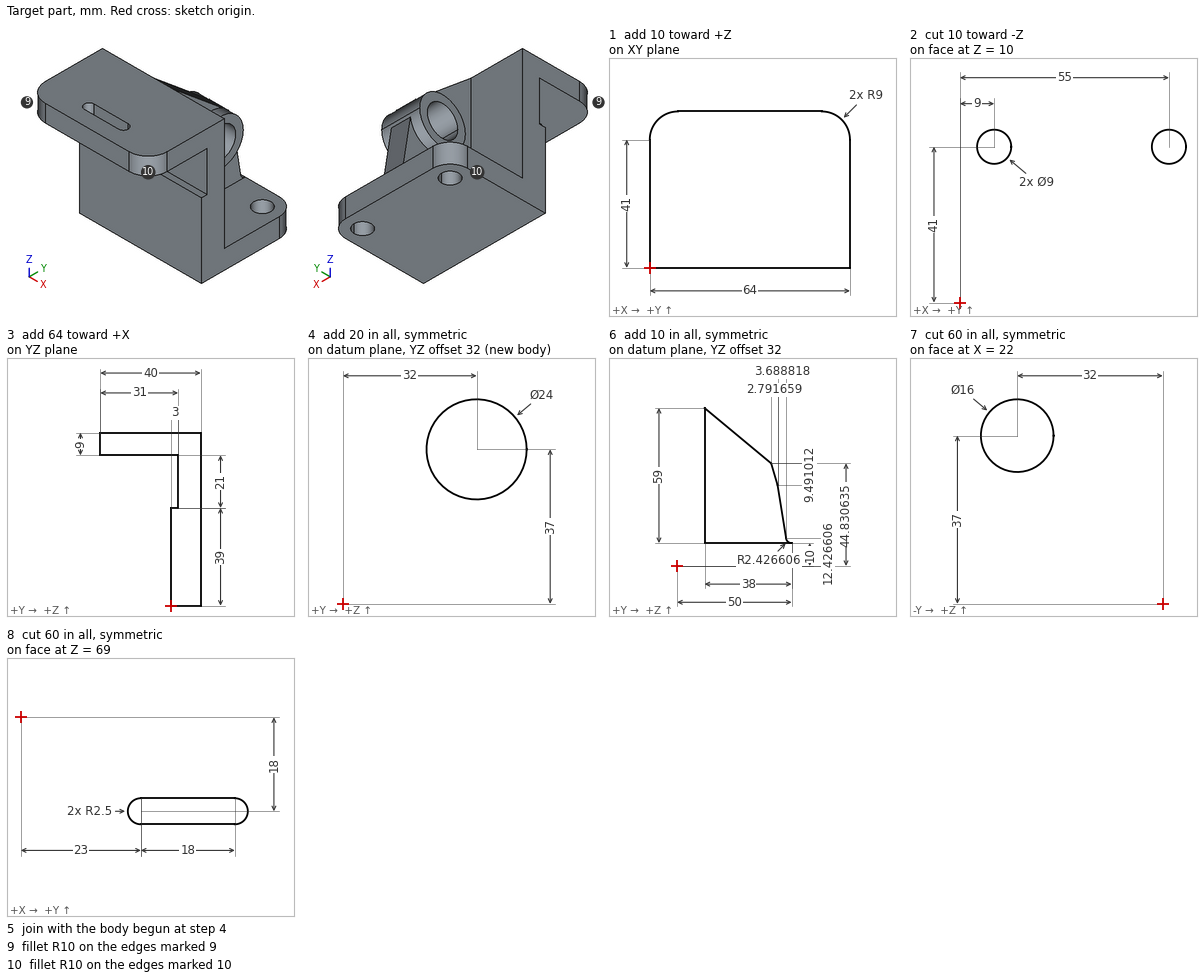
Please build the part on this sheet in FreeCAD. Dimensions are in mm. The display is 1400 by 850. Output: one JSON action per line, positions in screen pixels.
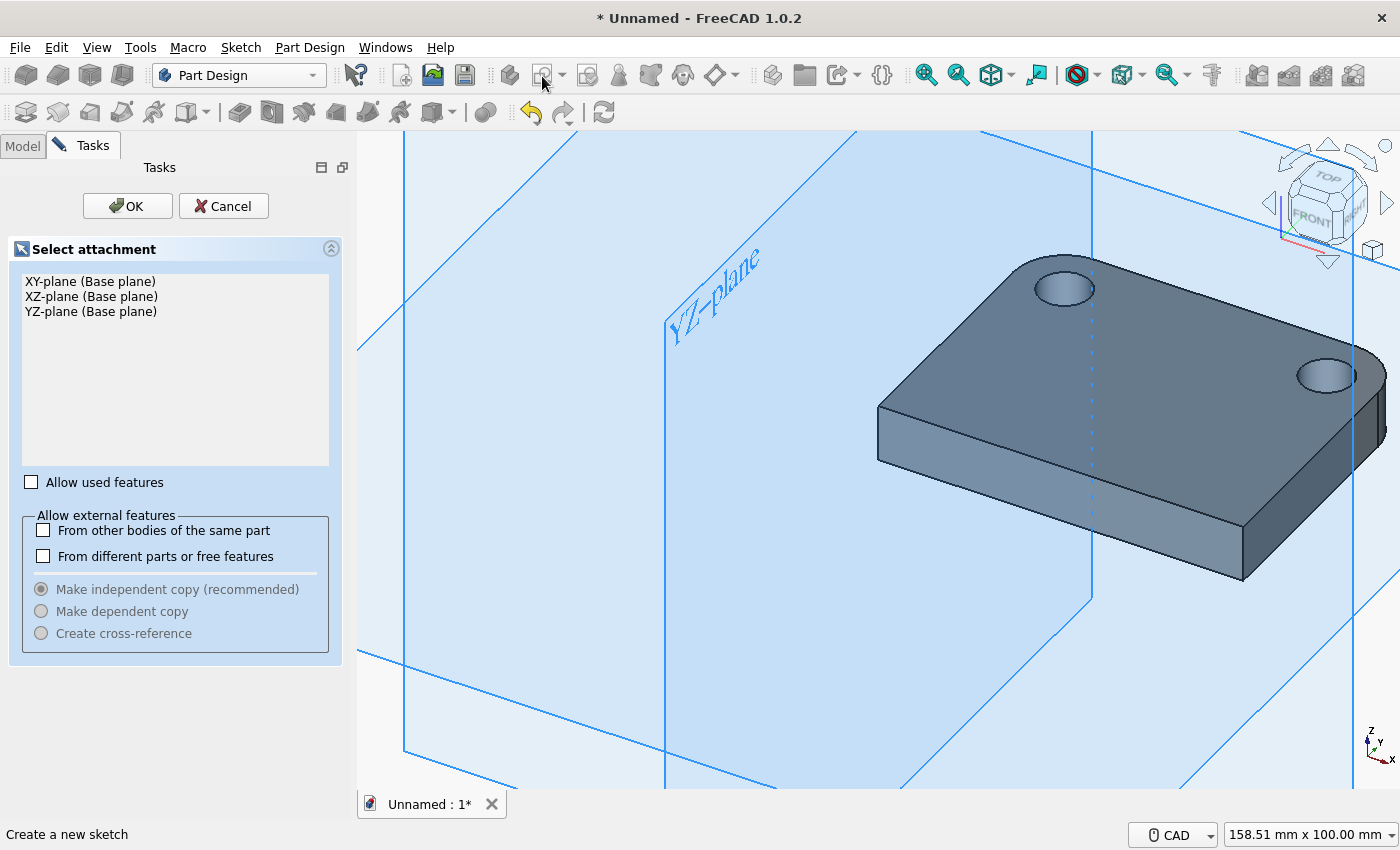
{"action": "left_click", "coordinate": [82, 312]}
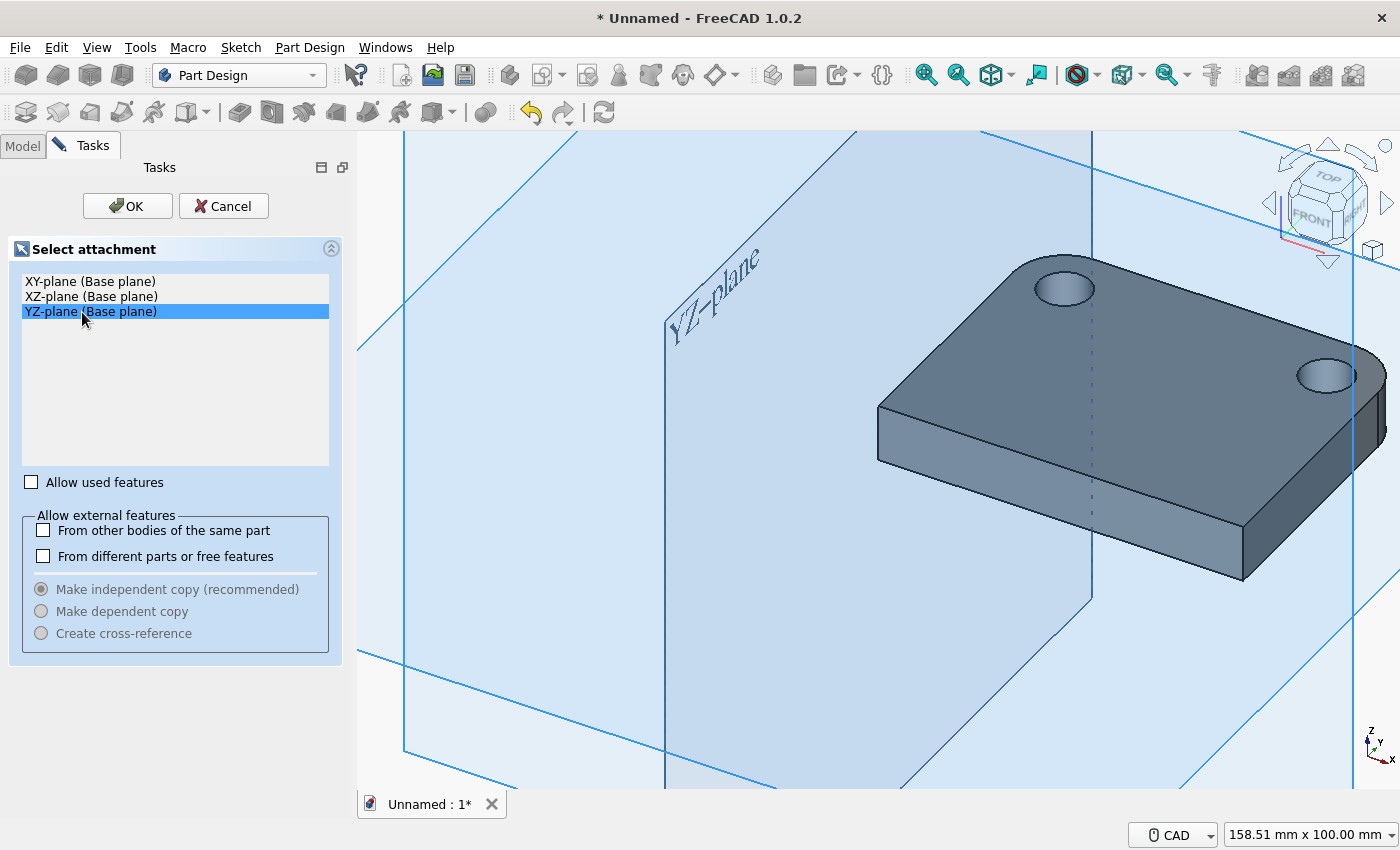
{"action": "left_click", "coordinate": [128, 206]}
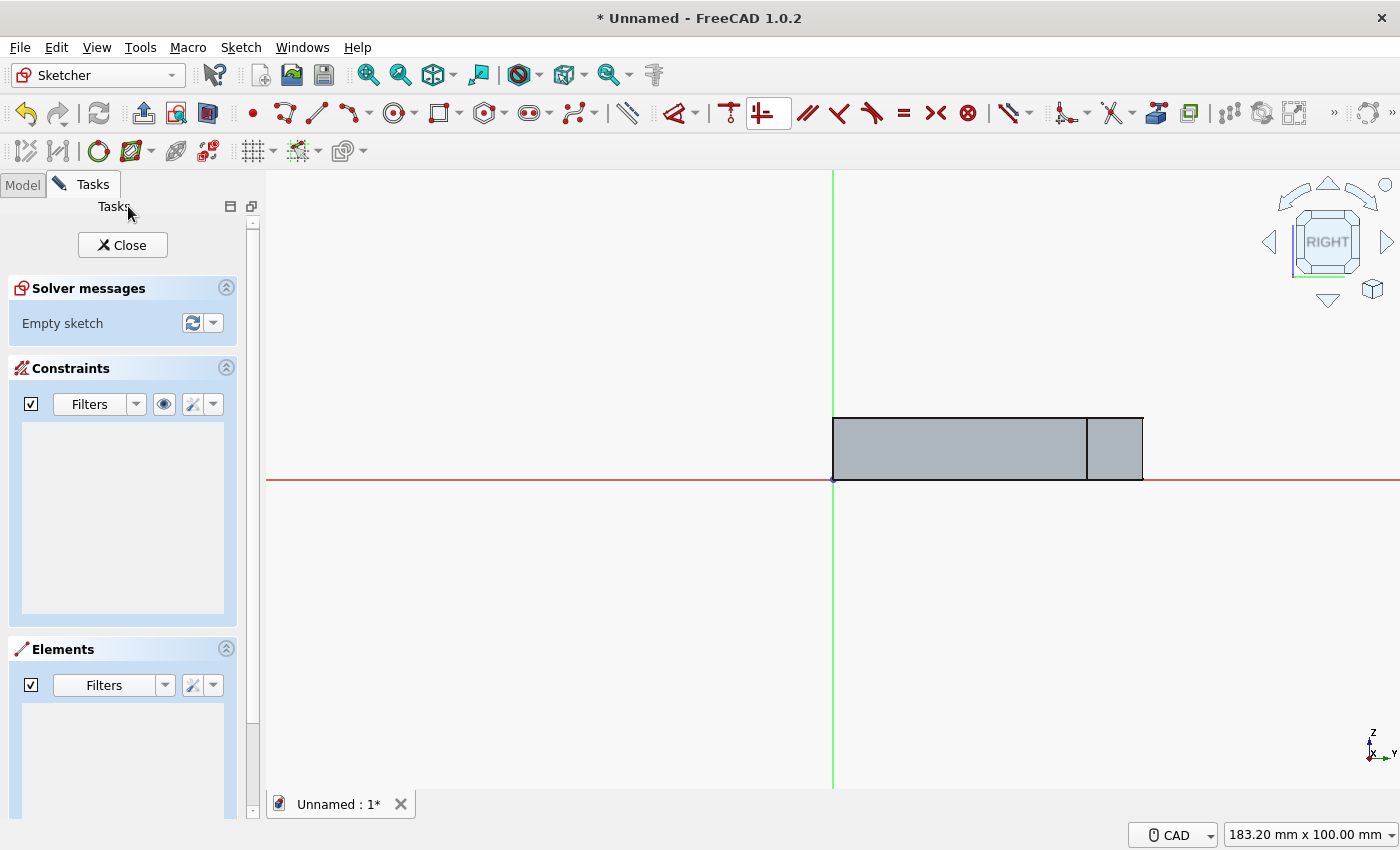
{"action": "left_click", "coordinate": [208, 114]}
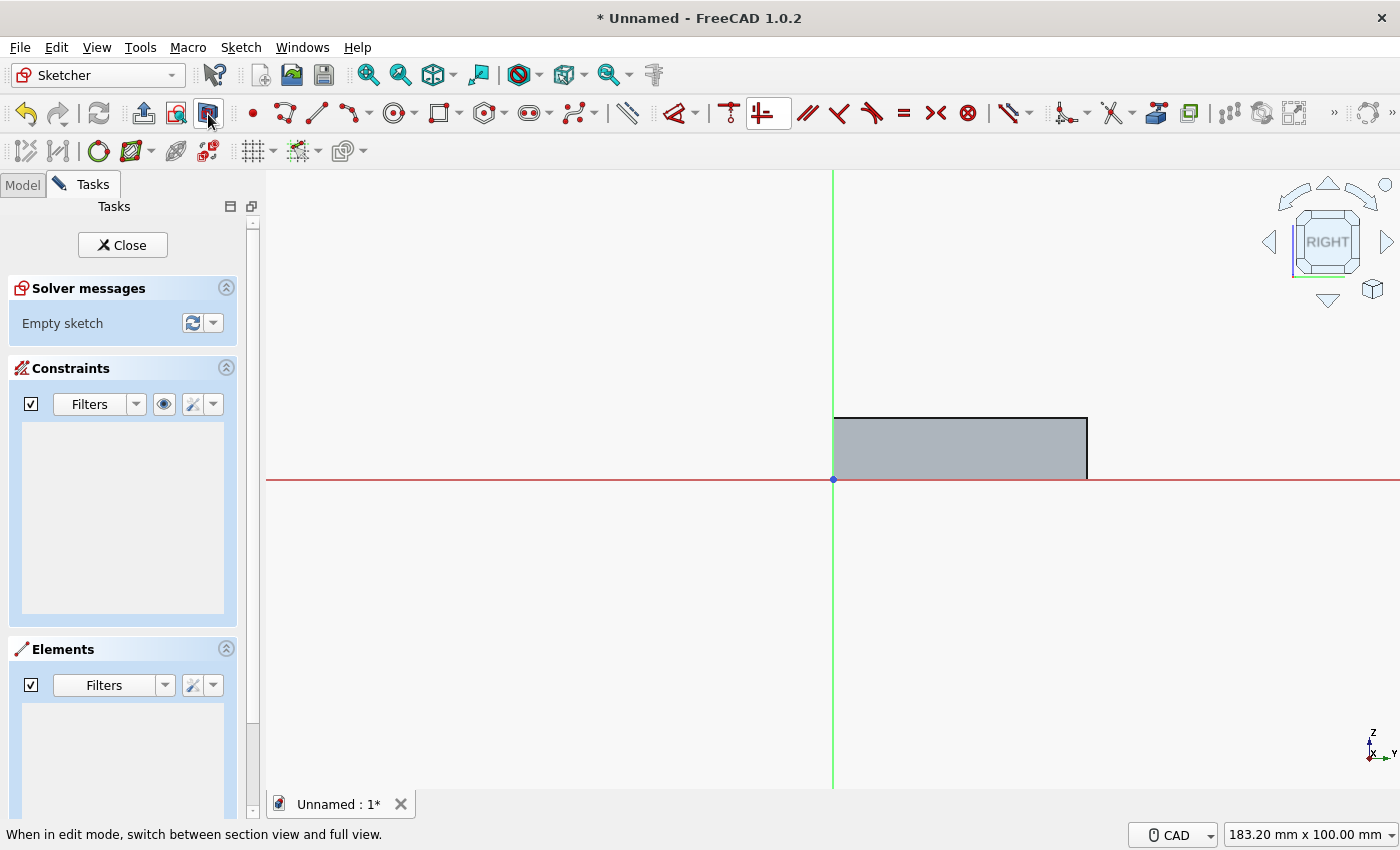
{"action": "scroll", "coordinate": [726, 761], "scroll_direction": "down", "scroll_amount": 2}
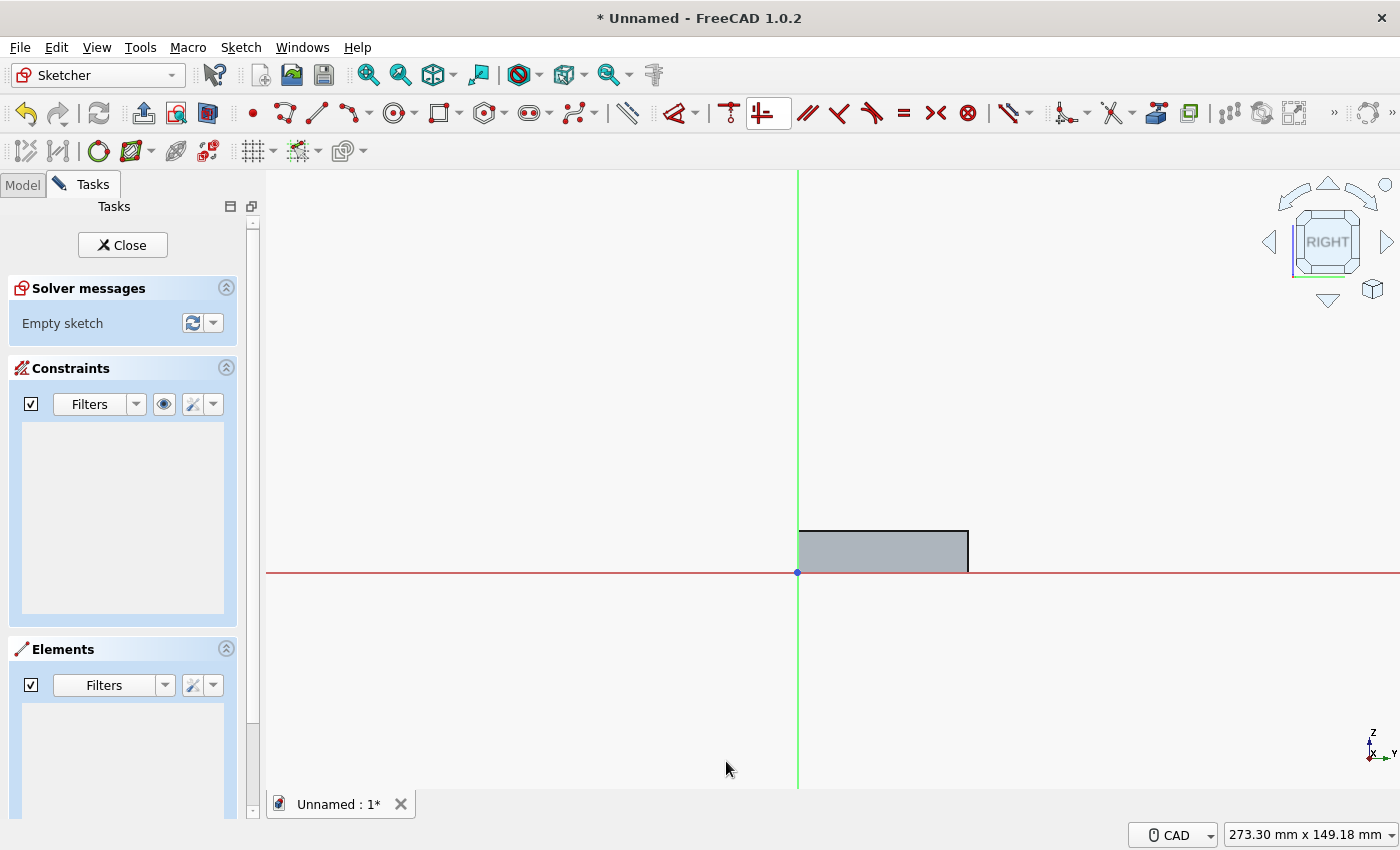
{"action": "scroll", "coordinate": [765, 328], "scroll_direction": "up", "scroll_amount": 2}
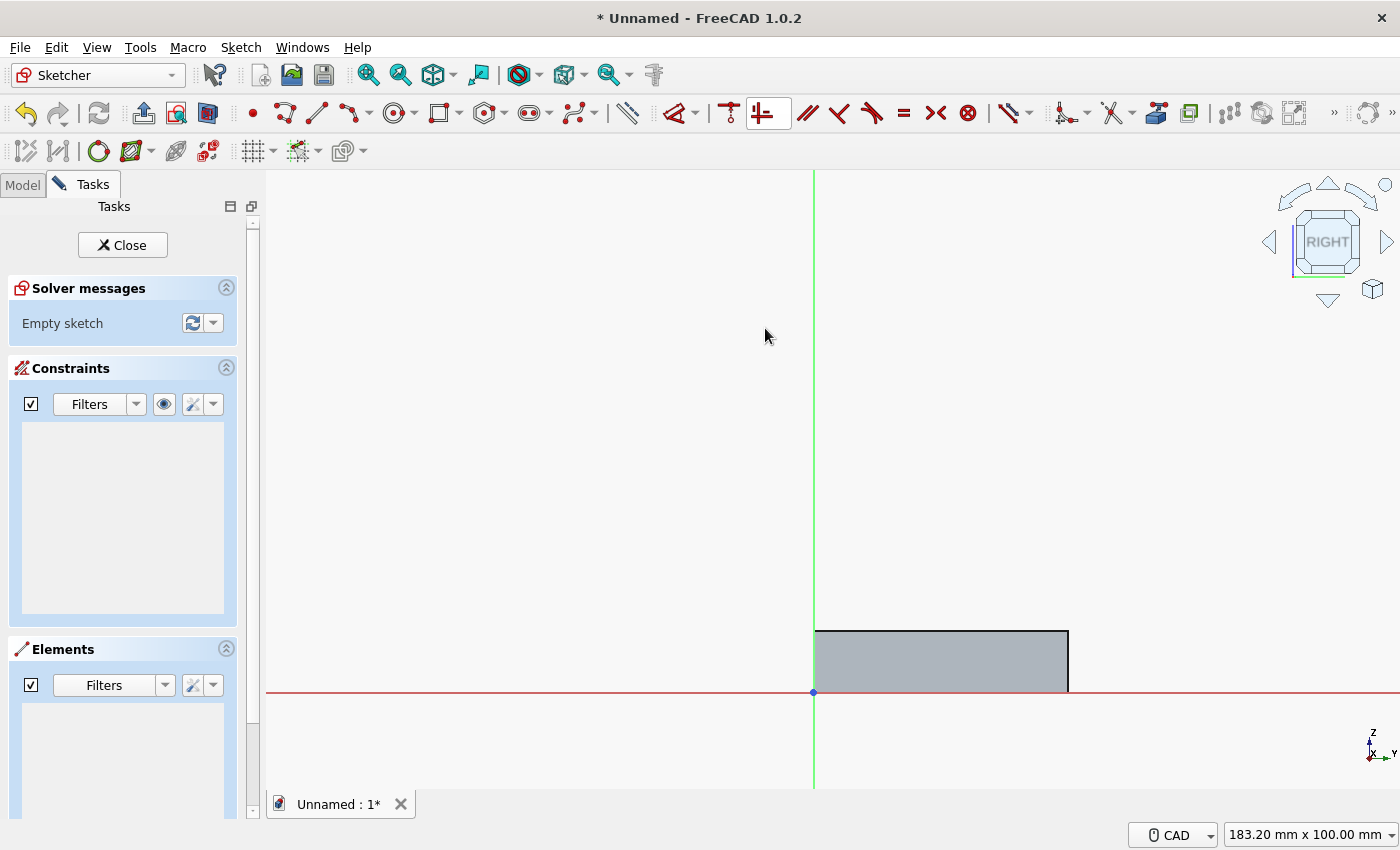
{"action": "left_click", "coordinate": [286, 114]}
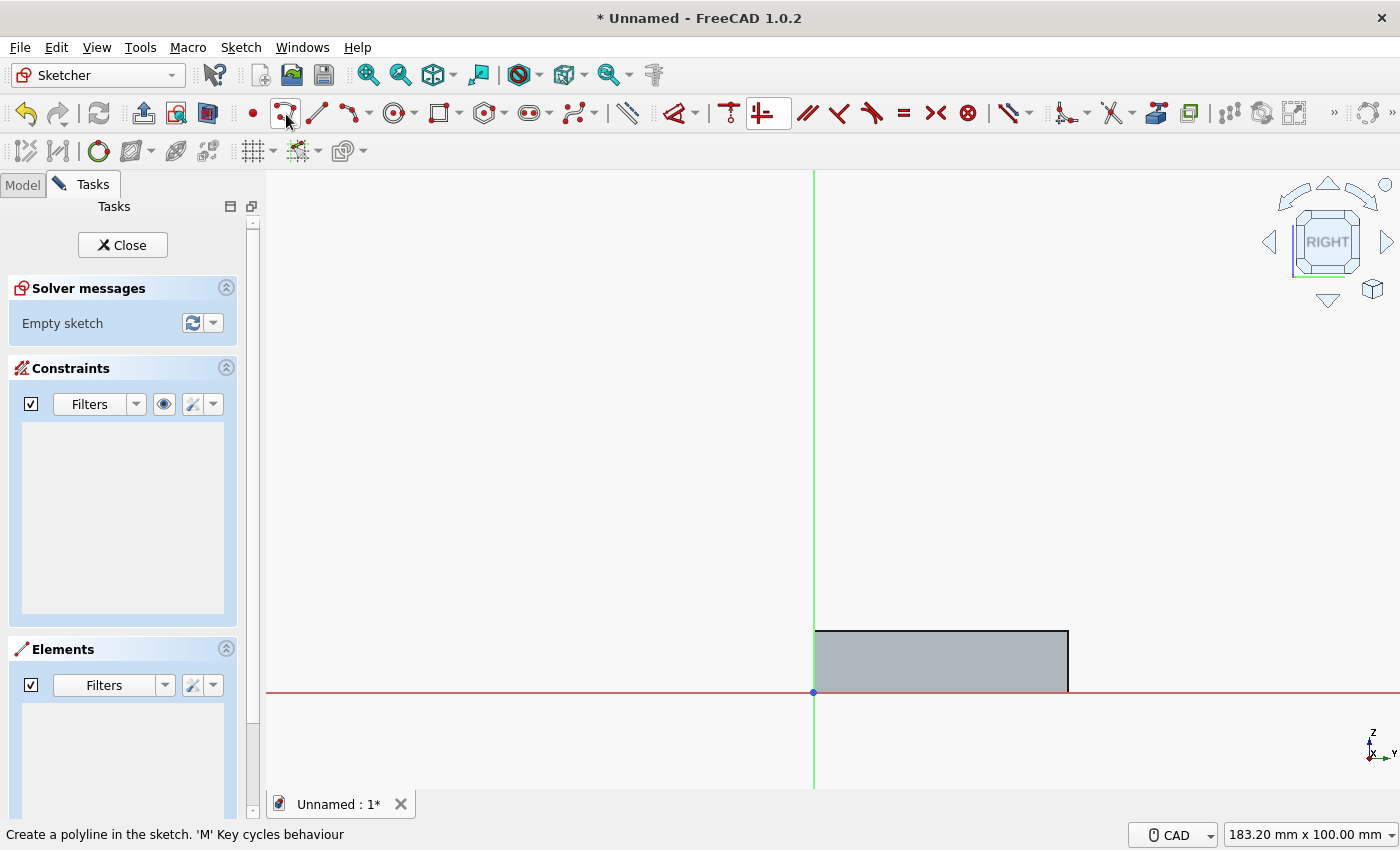
{"action": "left_click", "coordinate": [814, 693]}
{"action": "left_click", "coordinate": [805, 451]}
{"action": "left_click", "coordinate": [832, 451]}
{"action": "left_click", "coordinate": [832, 321]}
{"action": "left_click", "coordinate": [640, 321]}
{"action": "left_click", "coordinate": [640, 266]}
{"action": "left_click", "coordinate": [888, 266]}
{"action": "left_click", "coordinate": [888, 684]}
{"action": "left_click", "coordinate": [814, 693]}
{"action": "key", "text": "Escape"}
{"action": "key", "text": "Escape"}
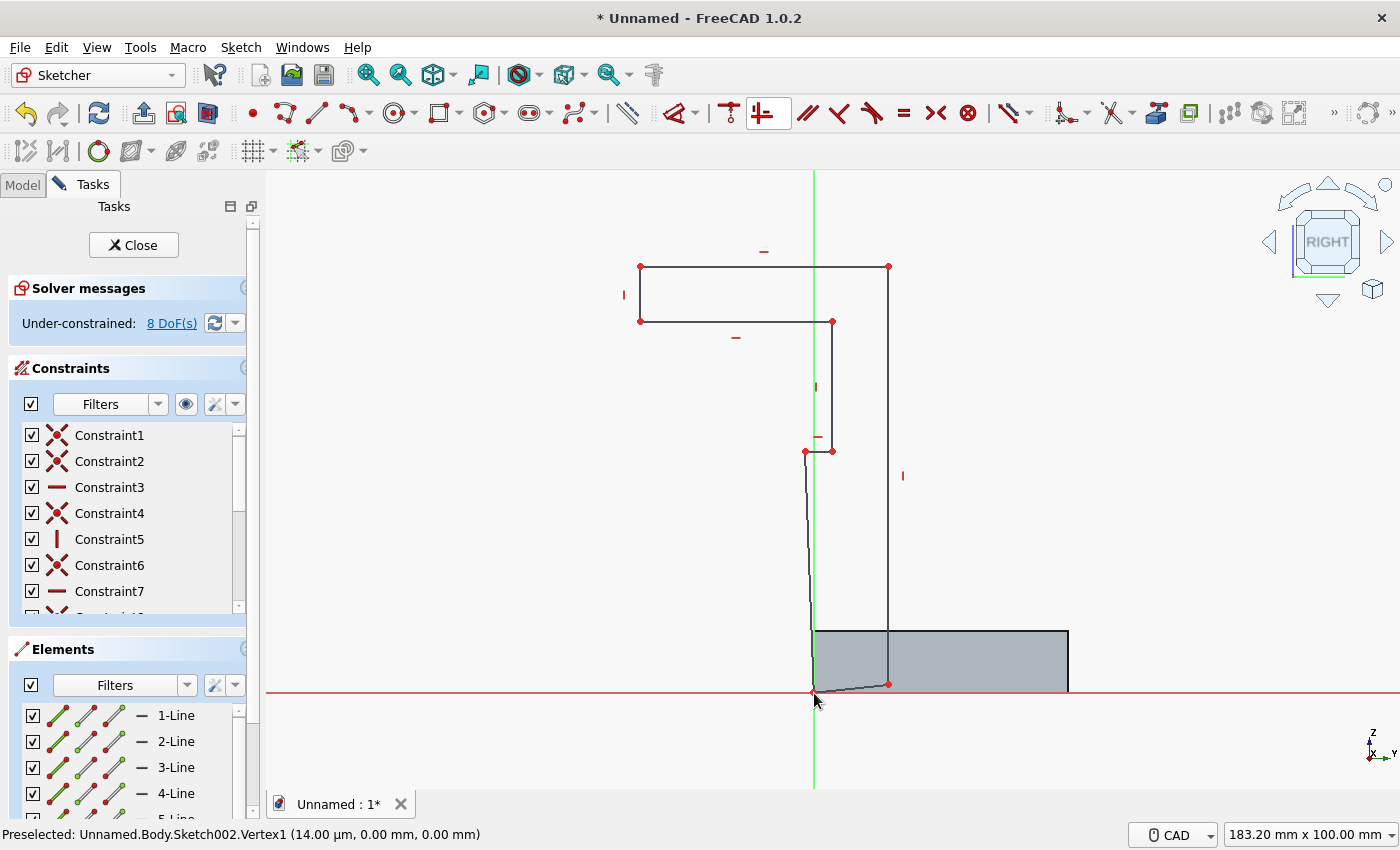
{"action": "left_click", "coordinate": [811, 621]}